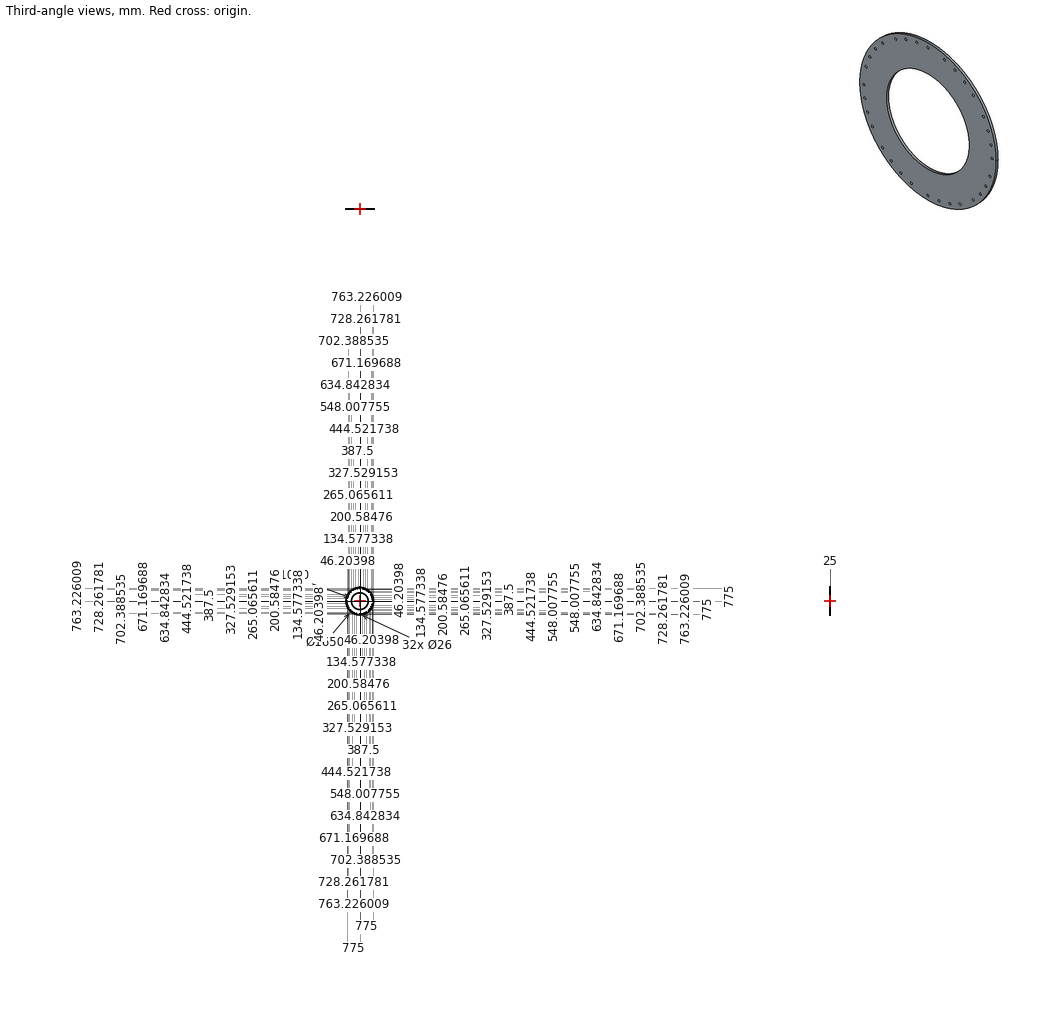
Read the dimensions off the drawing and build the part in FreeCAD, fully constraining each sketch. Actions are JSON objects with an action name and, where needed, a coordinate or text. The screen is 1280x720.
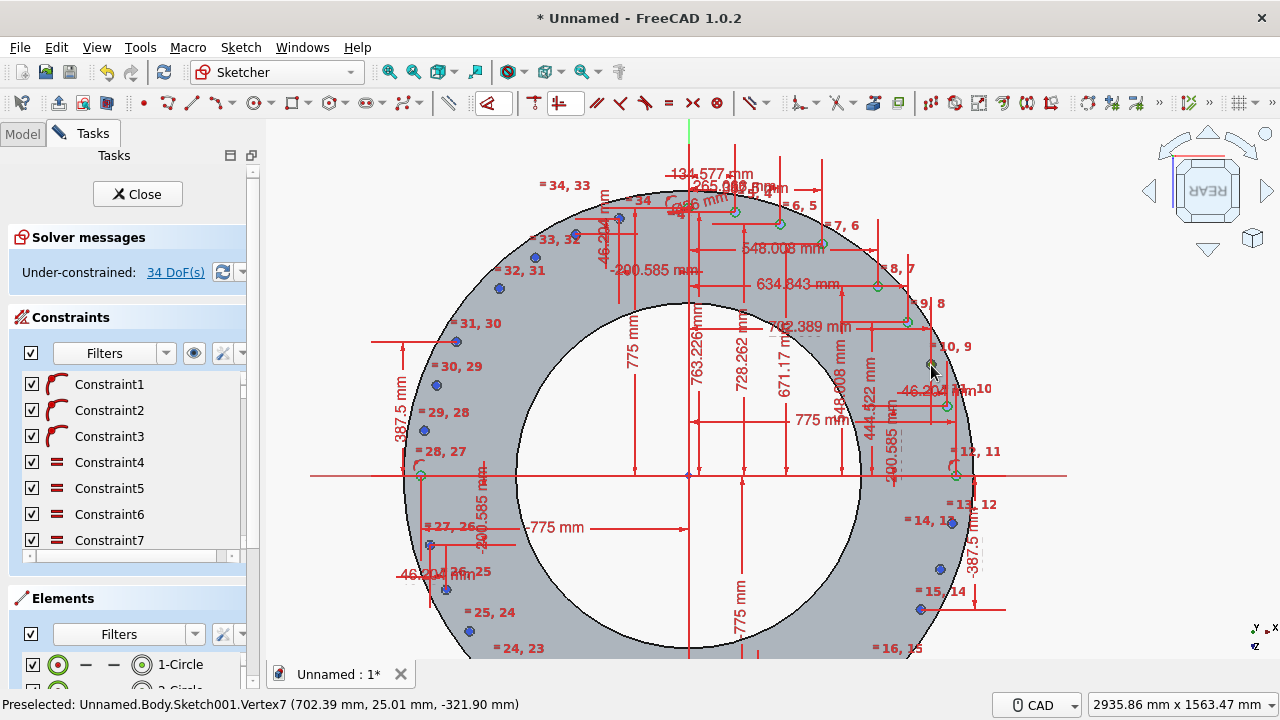
{"action": "key", "text": "i"}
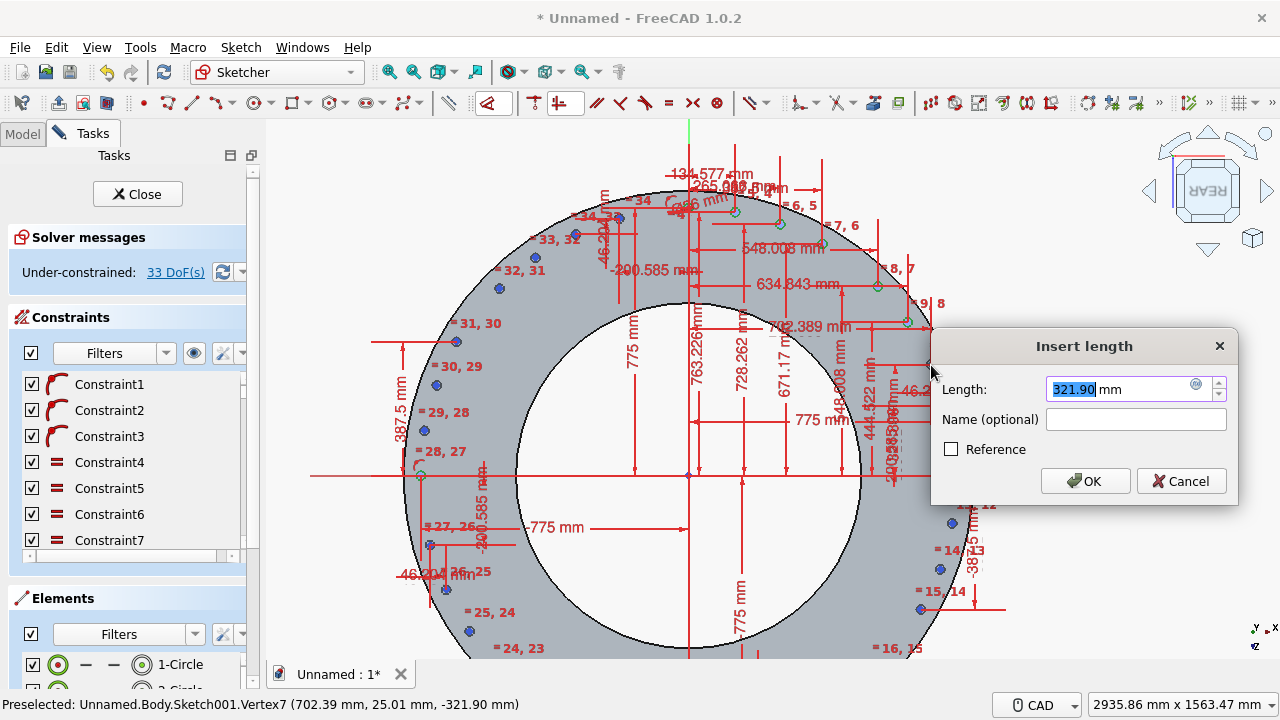
{"action": "type", "text": "327.529153"}
{"action": "key", "text": "Return"}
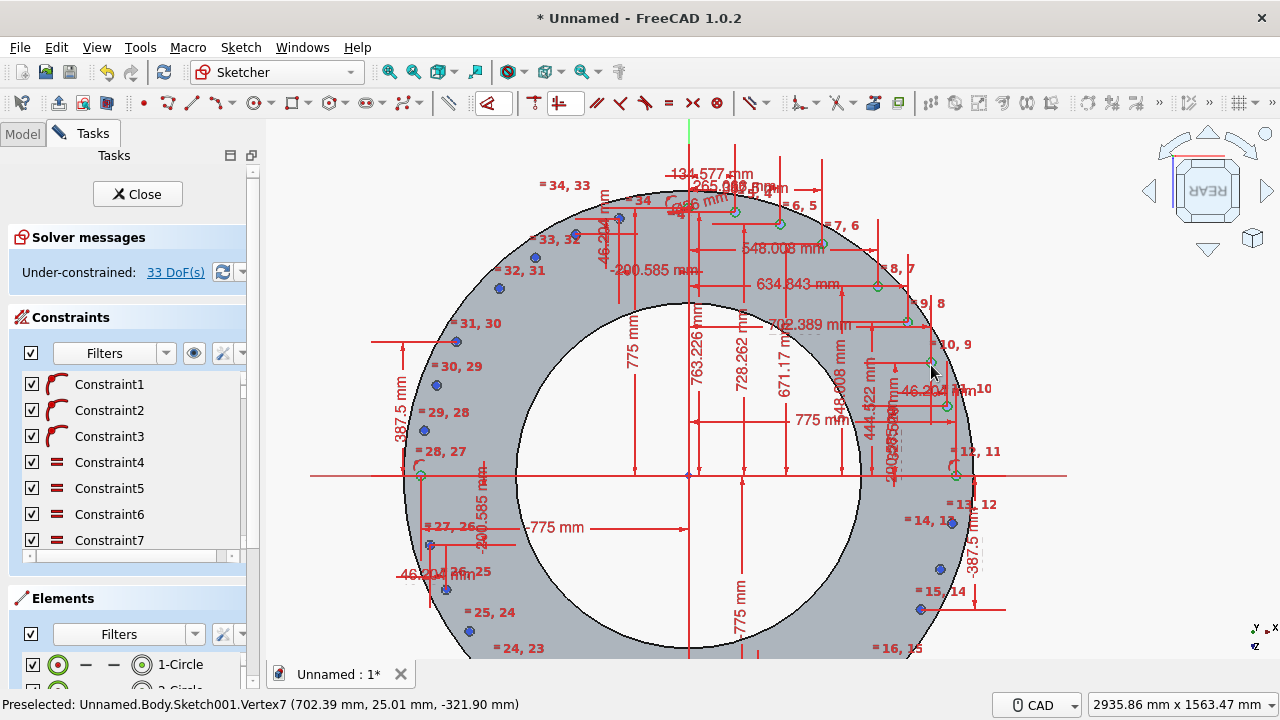
{"action": "left_click", "coordinate": [952, 523]}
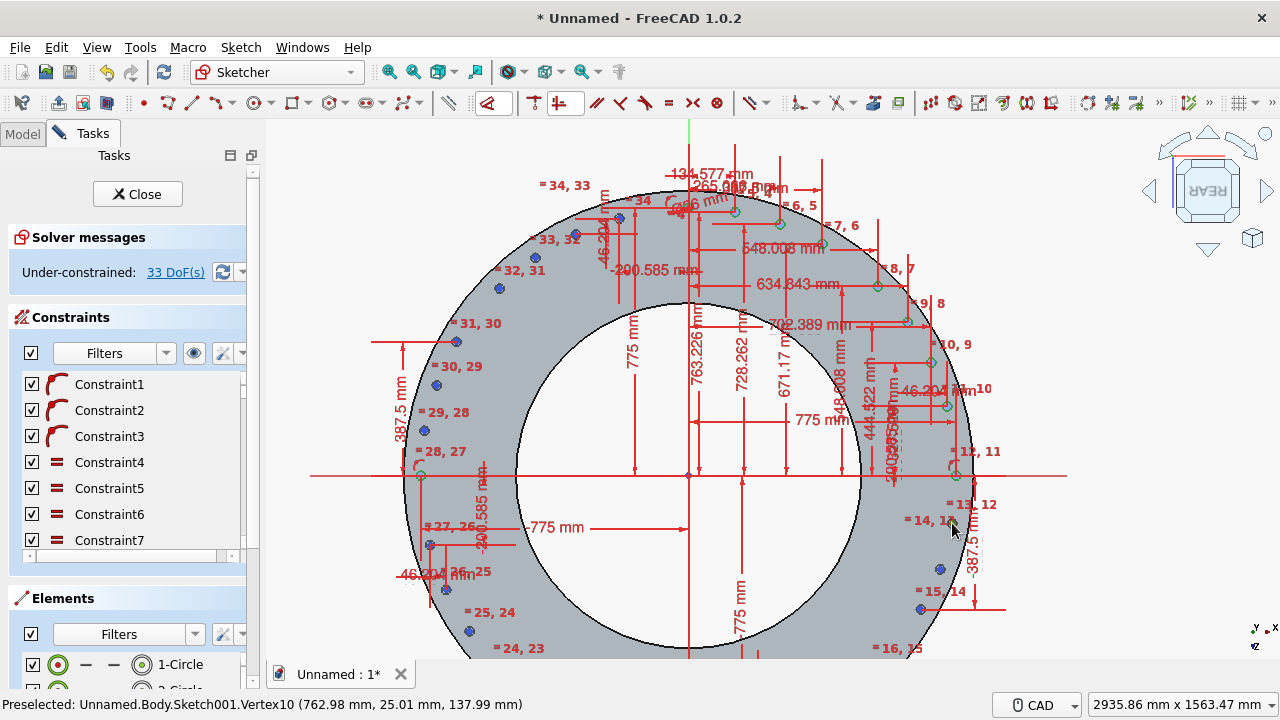
{"action": "key", "text": "l"}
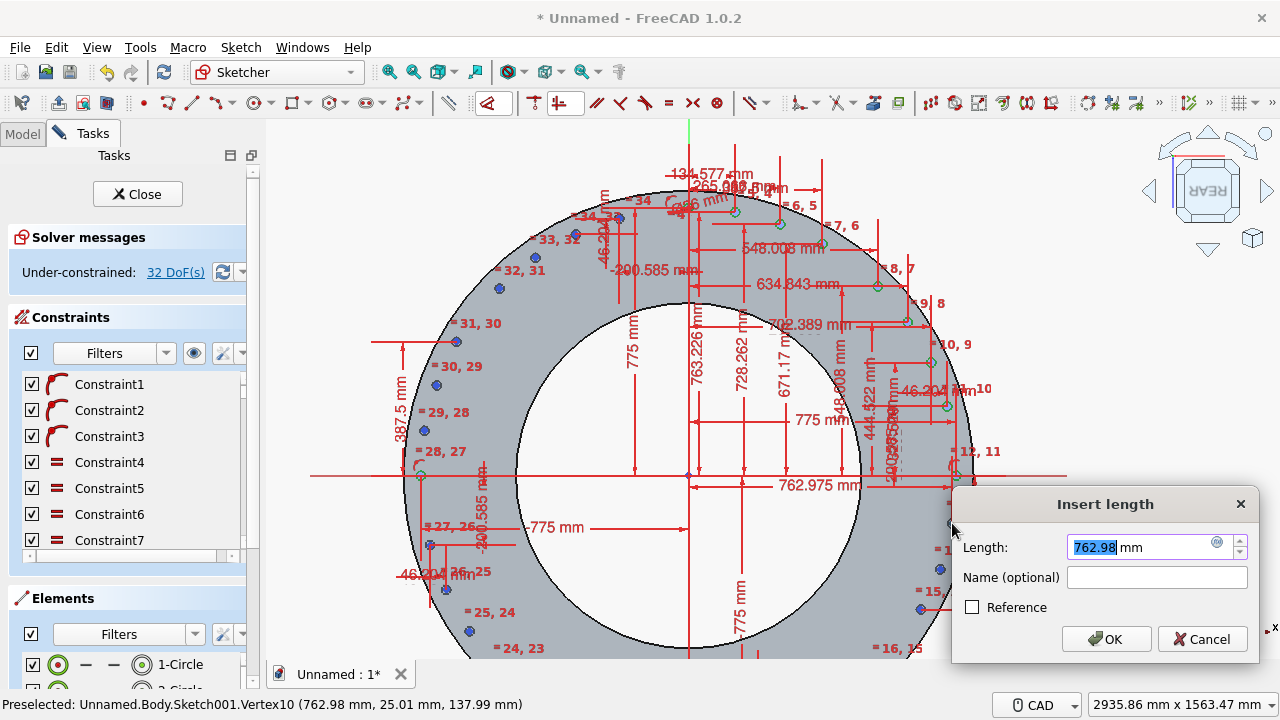
{"action": "type", "text": "763.226009"}
{"action": "key", "text": "Return"}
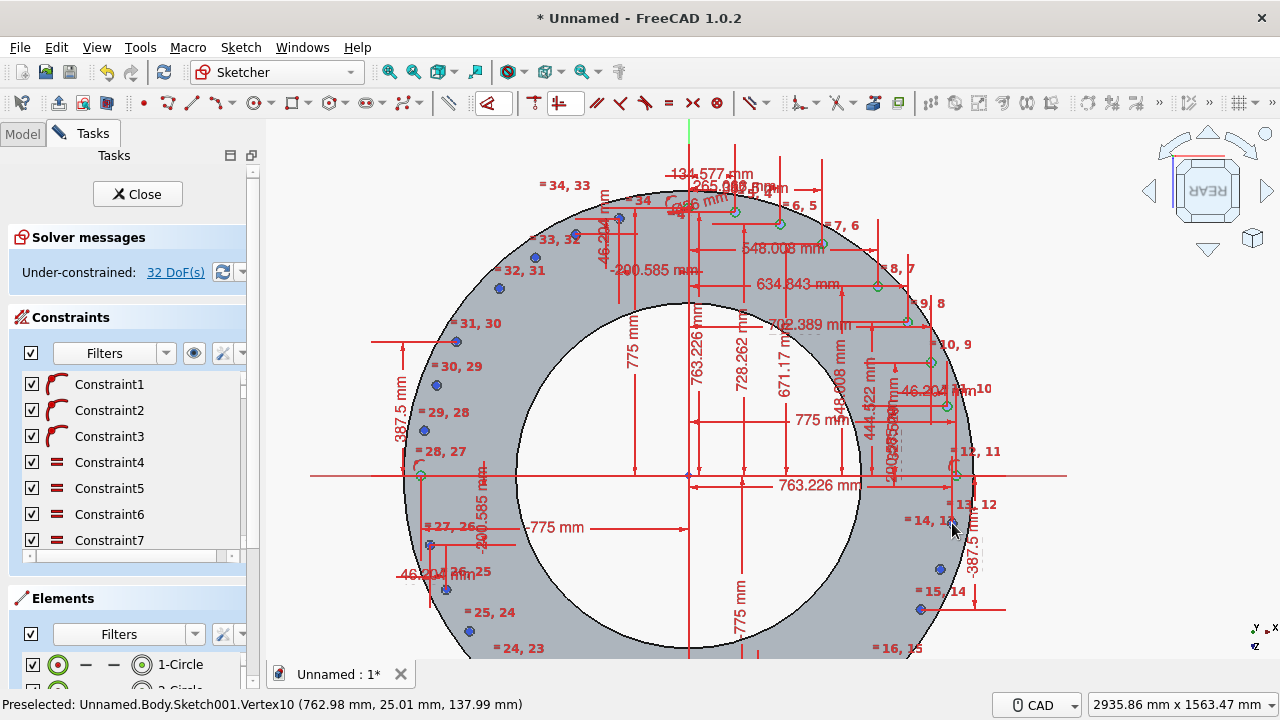
{"action": "left_click", "coordinate": [952, 523]}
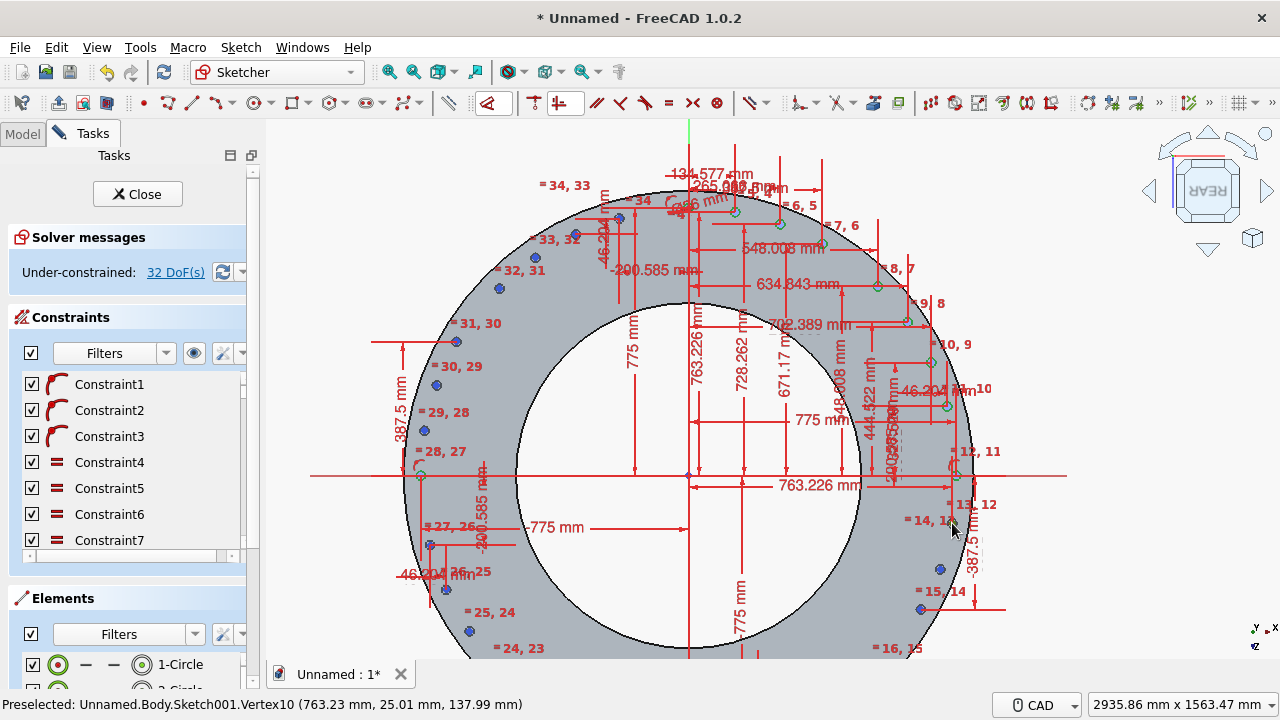
{"action": "left_click", "coordinate": [506, 104]}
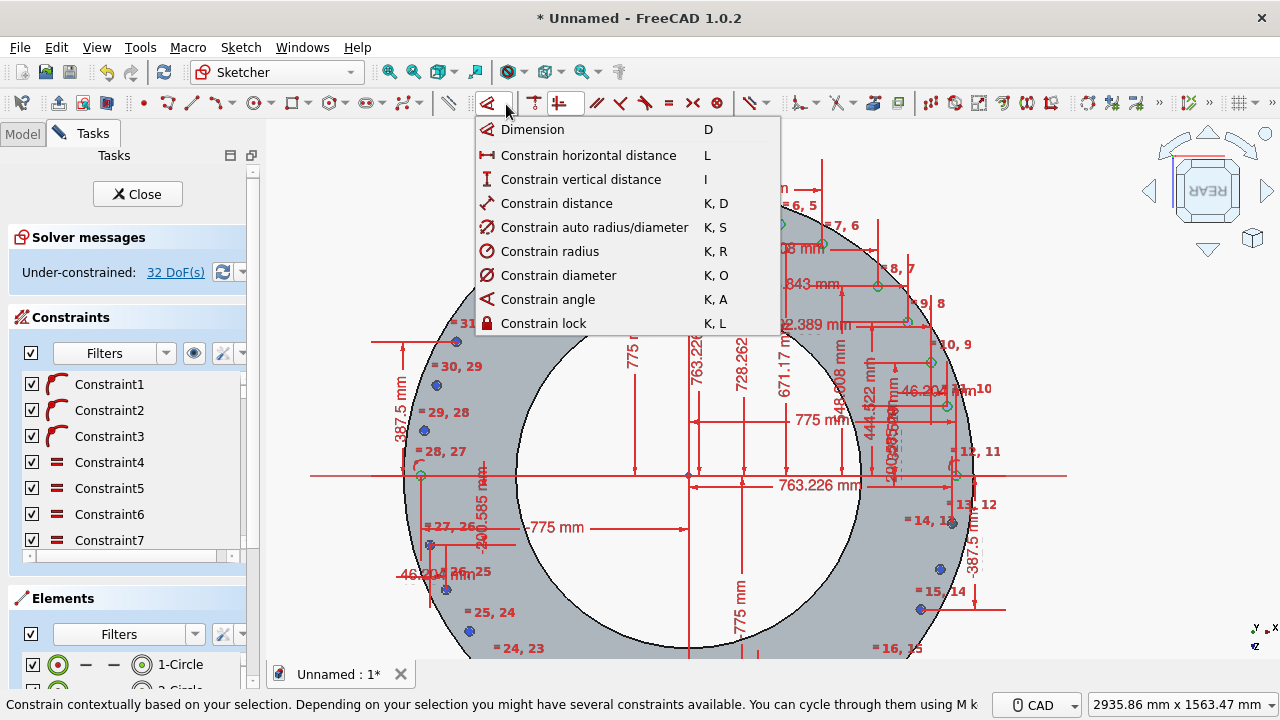
{"action": "left_click", "coordinate": [628, 179]}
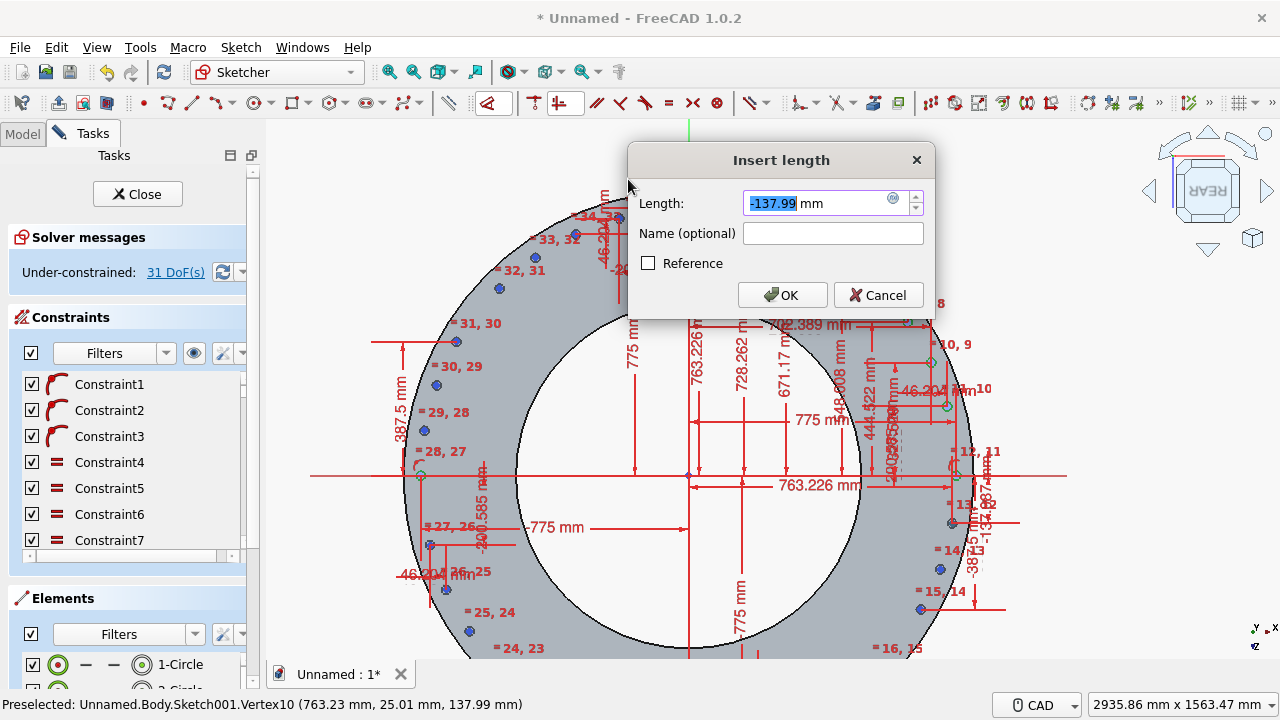
{"action": "type", "text": "-134.577338"}
{"action": "key", "text": "Return"}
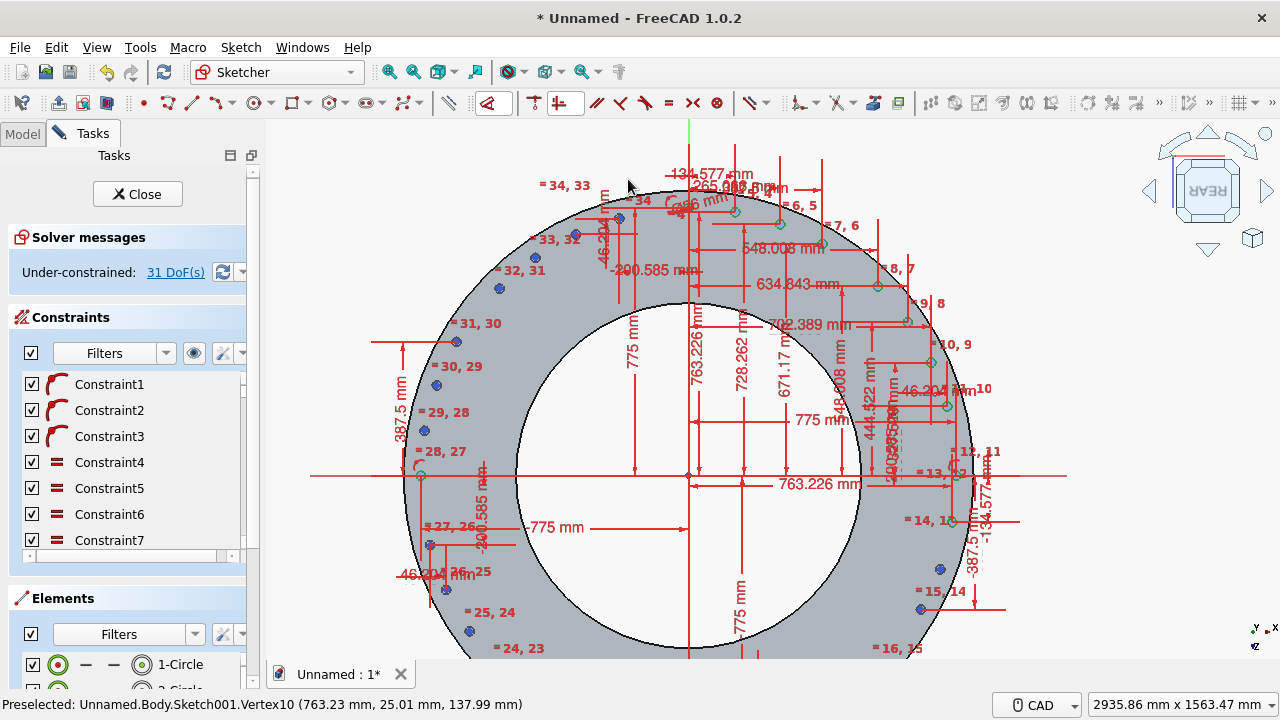
{"action": "left_click", "coordinate": [940, 569]}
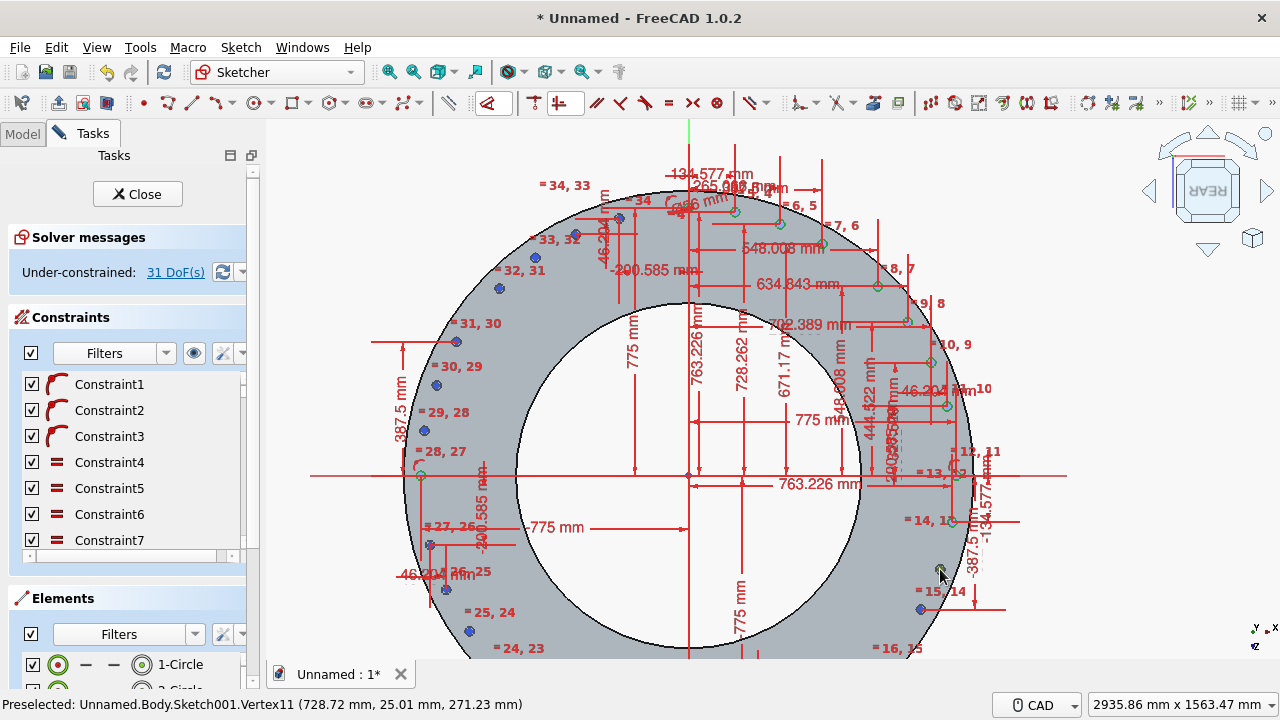
{"action": "key", "text": "l"}